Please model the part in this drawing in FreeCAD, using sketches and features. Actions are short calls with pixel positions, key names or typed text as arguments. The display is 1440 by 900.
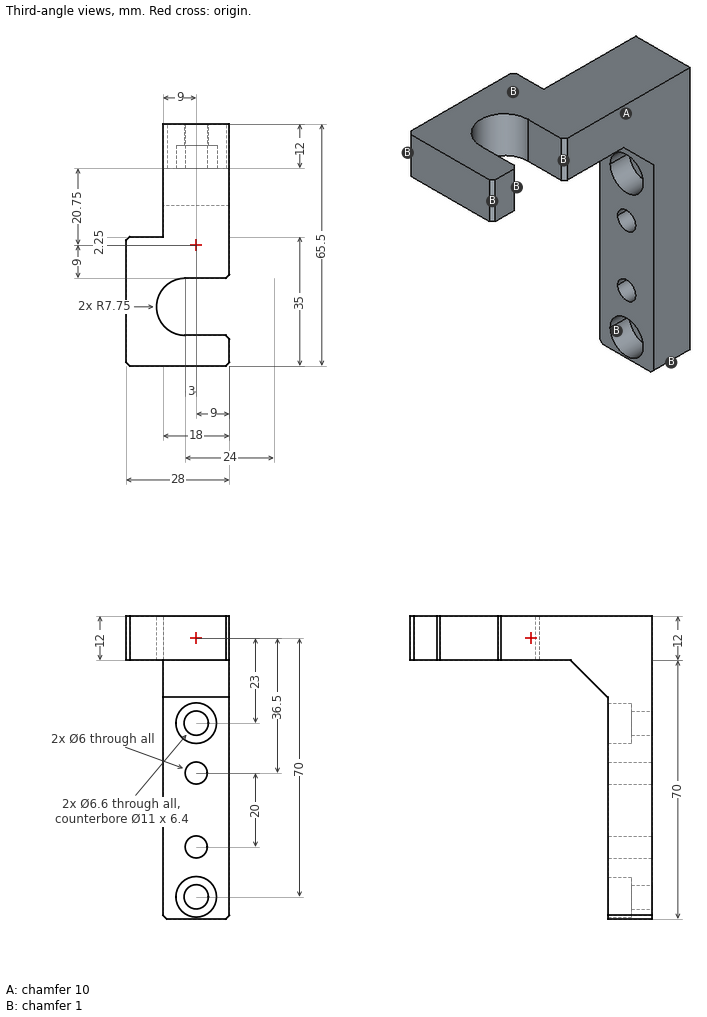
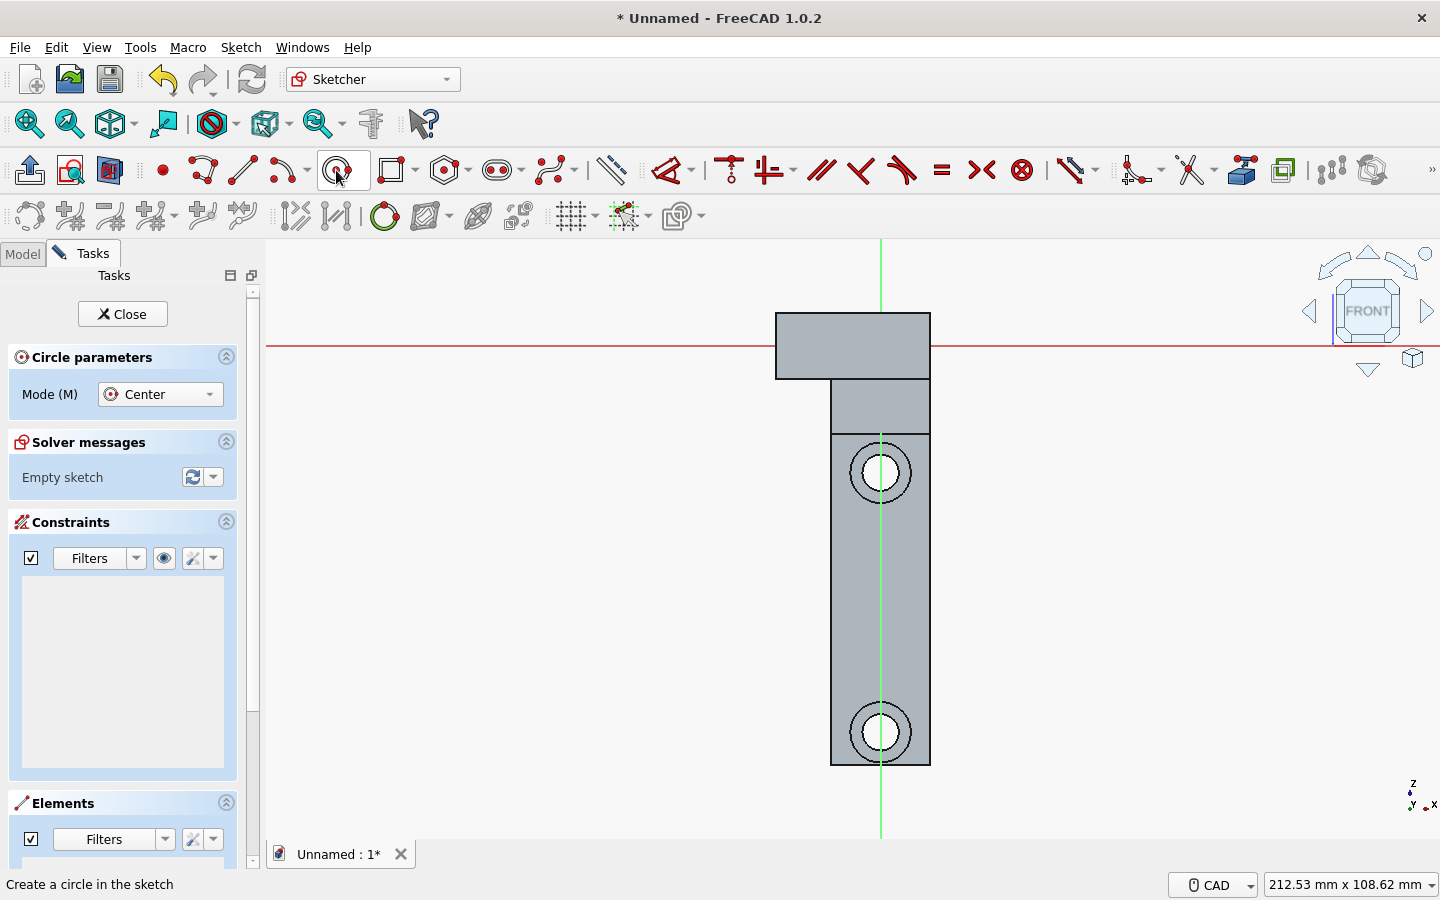
scroll(881, 547, up, 2)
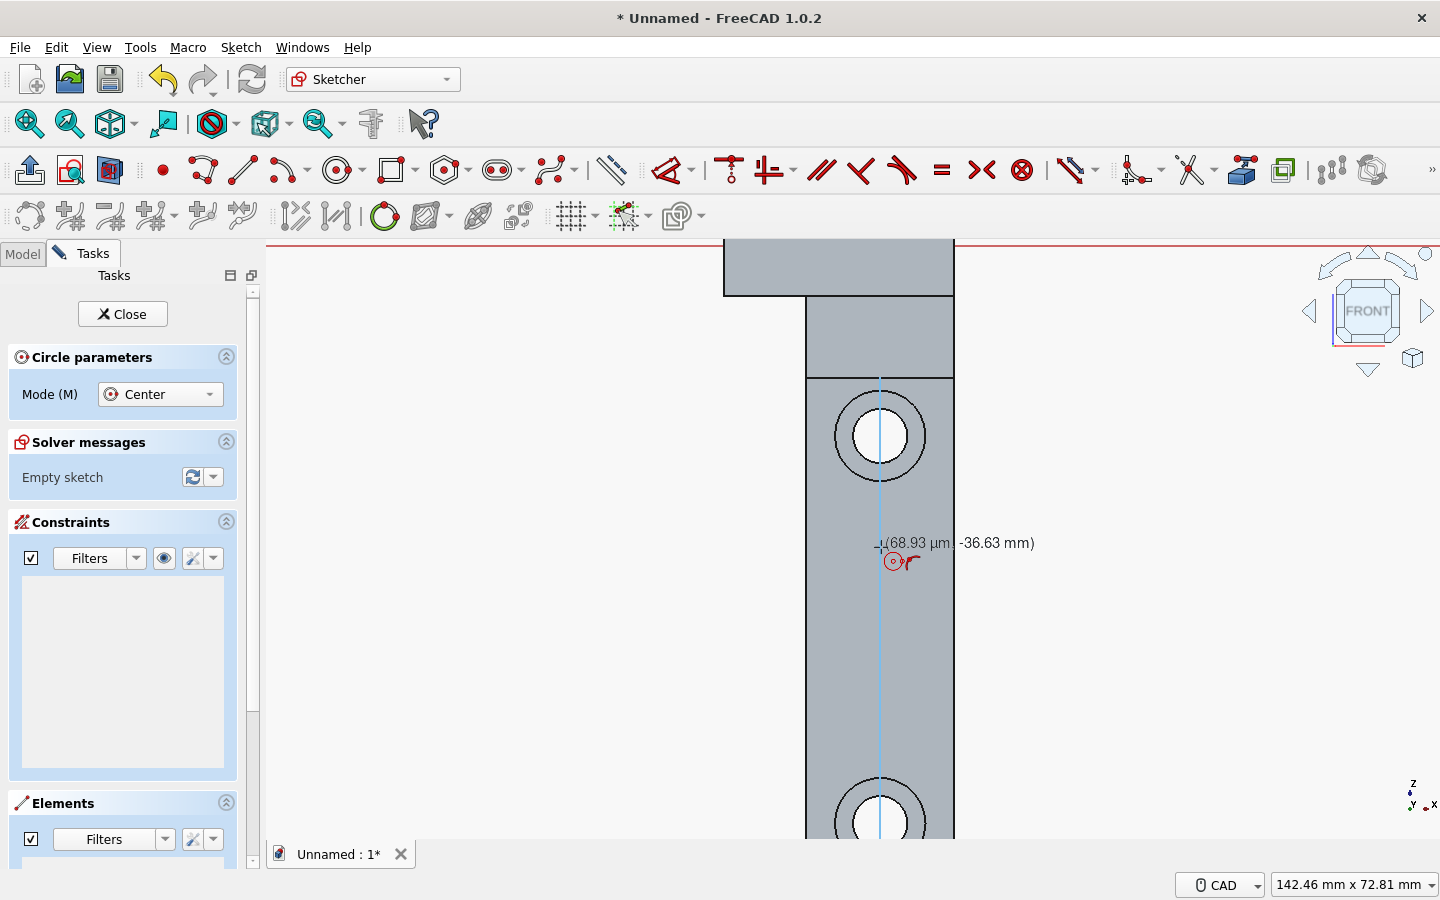
click(880, 547)
move(898, 530)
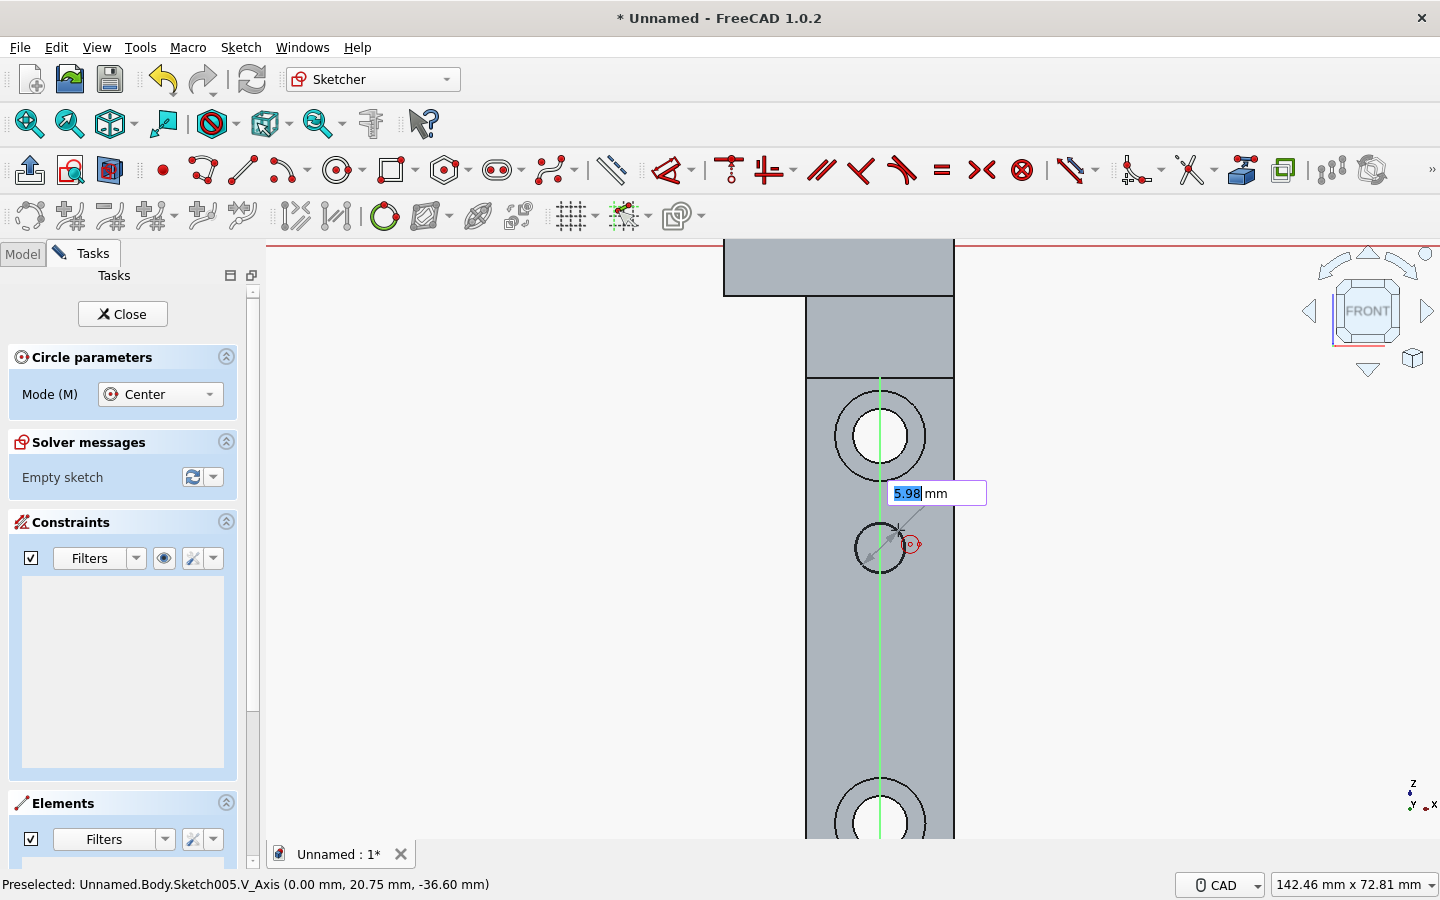
text(6)
key(Return)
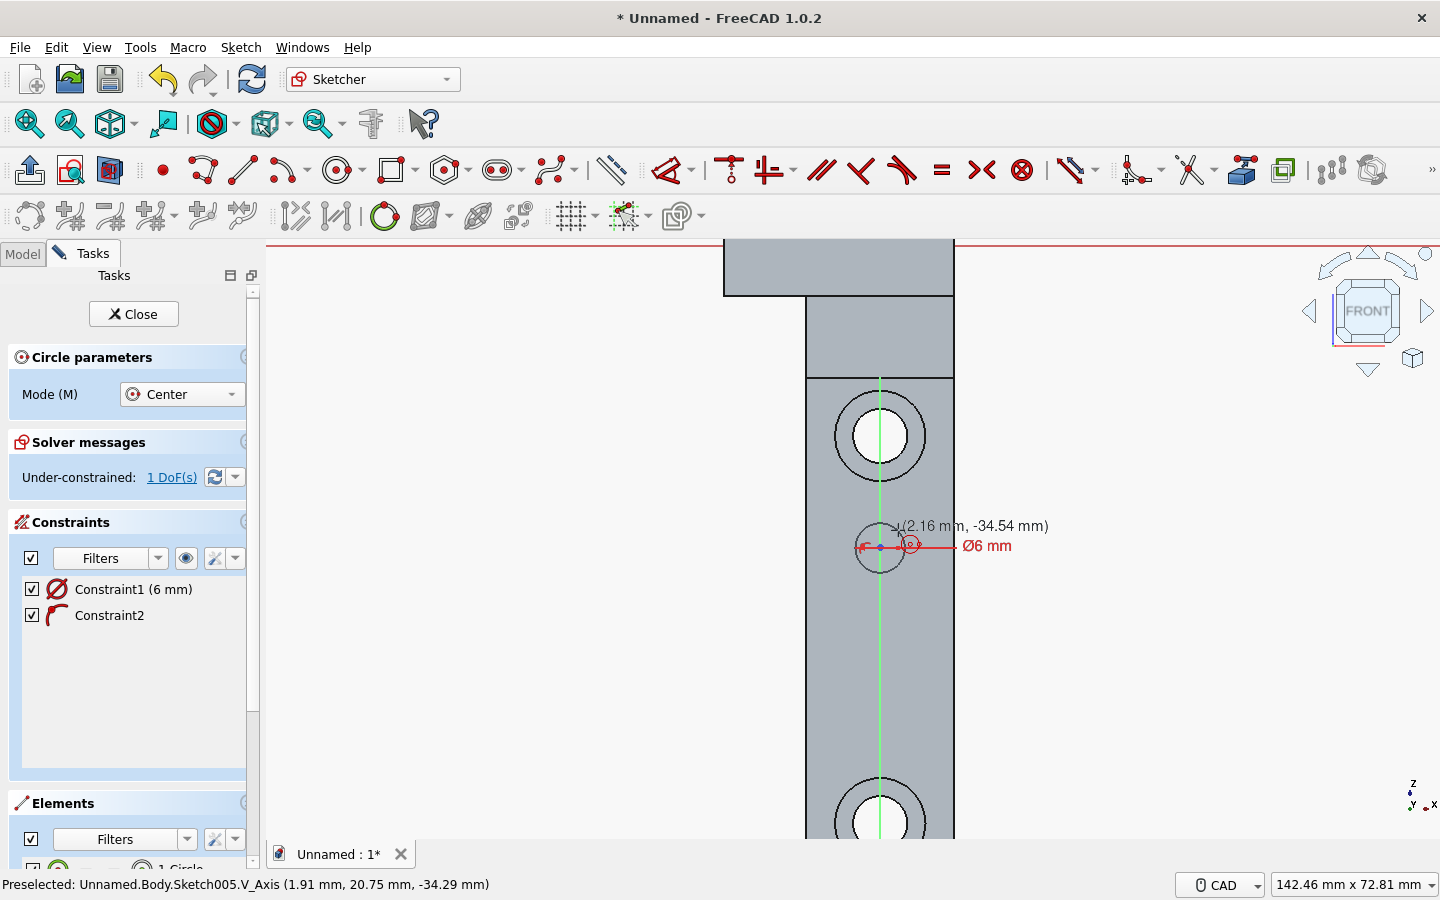
click(880, 712)
move(898, 695)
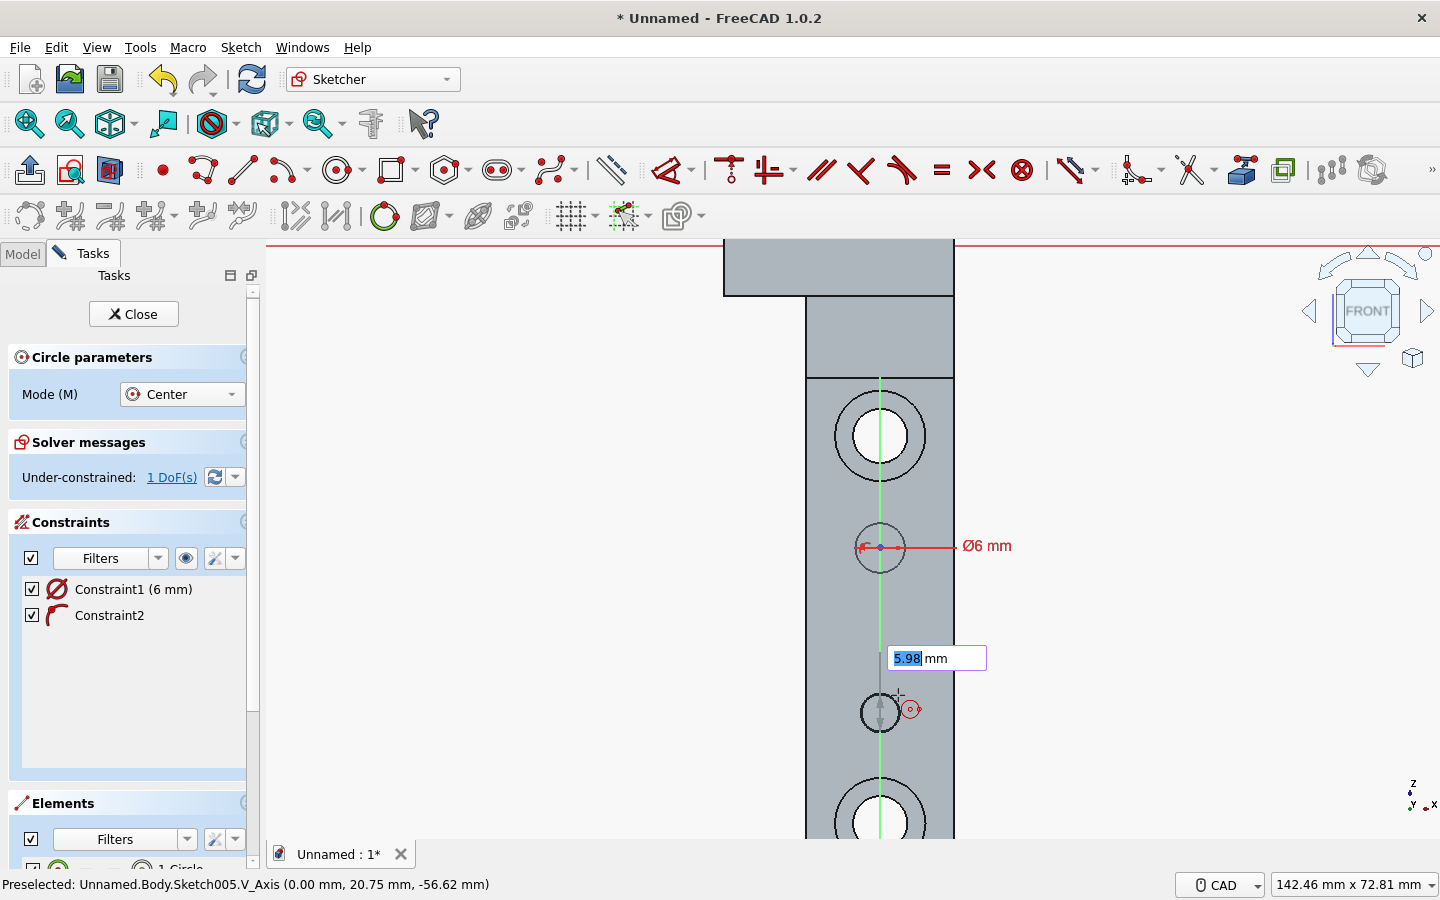
text(6)
key(Return)
key(Escape)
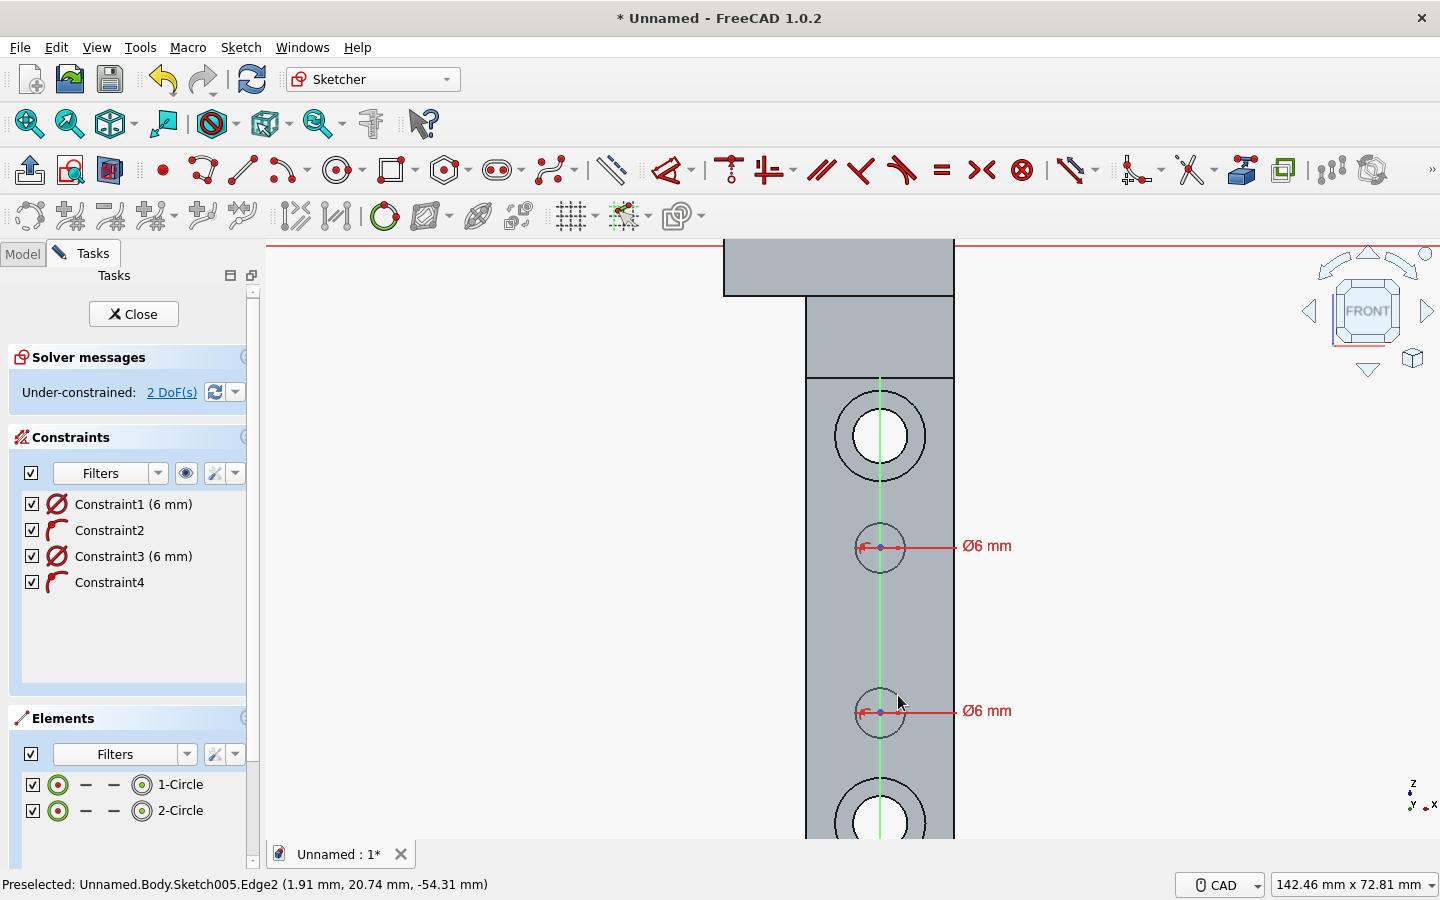
click(666, 170)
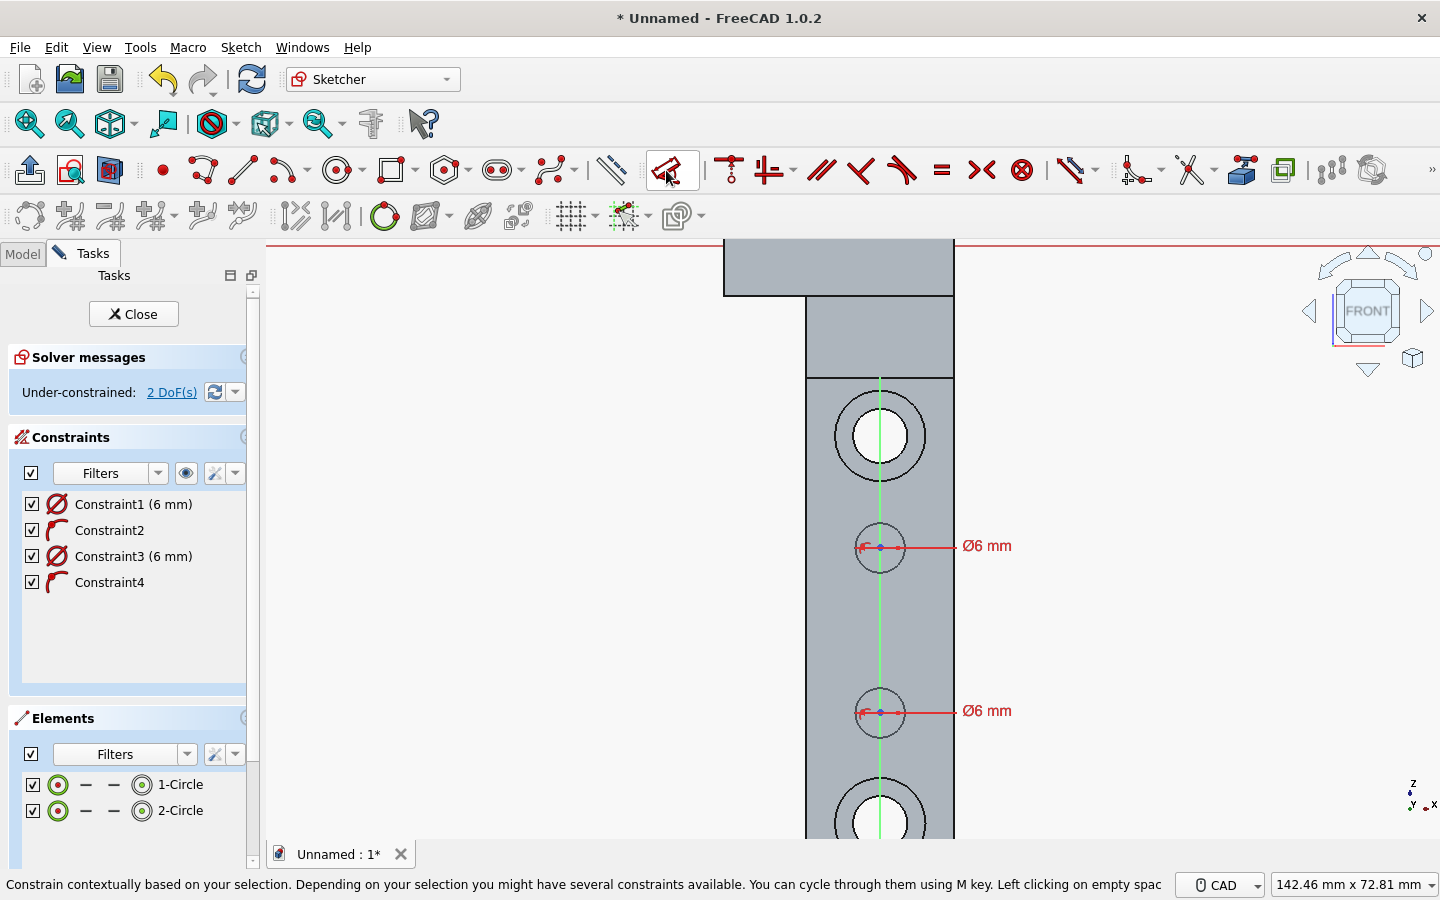
click(880, 548)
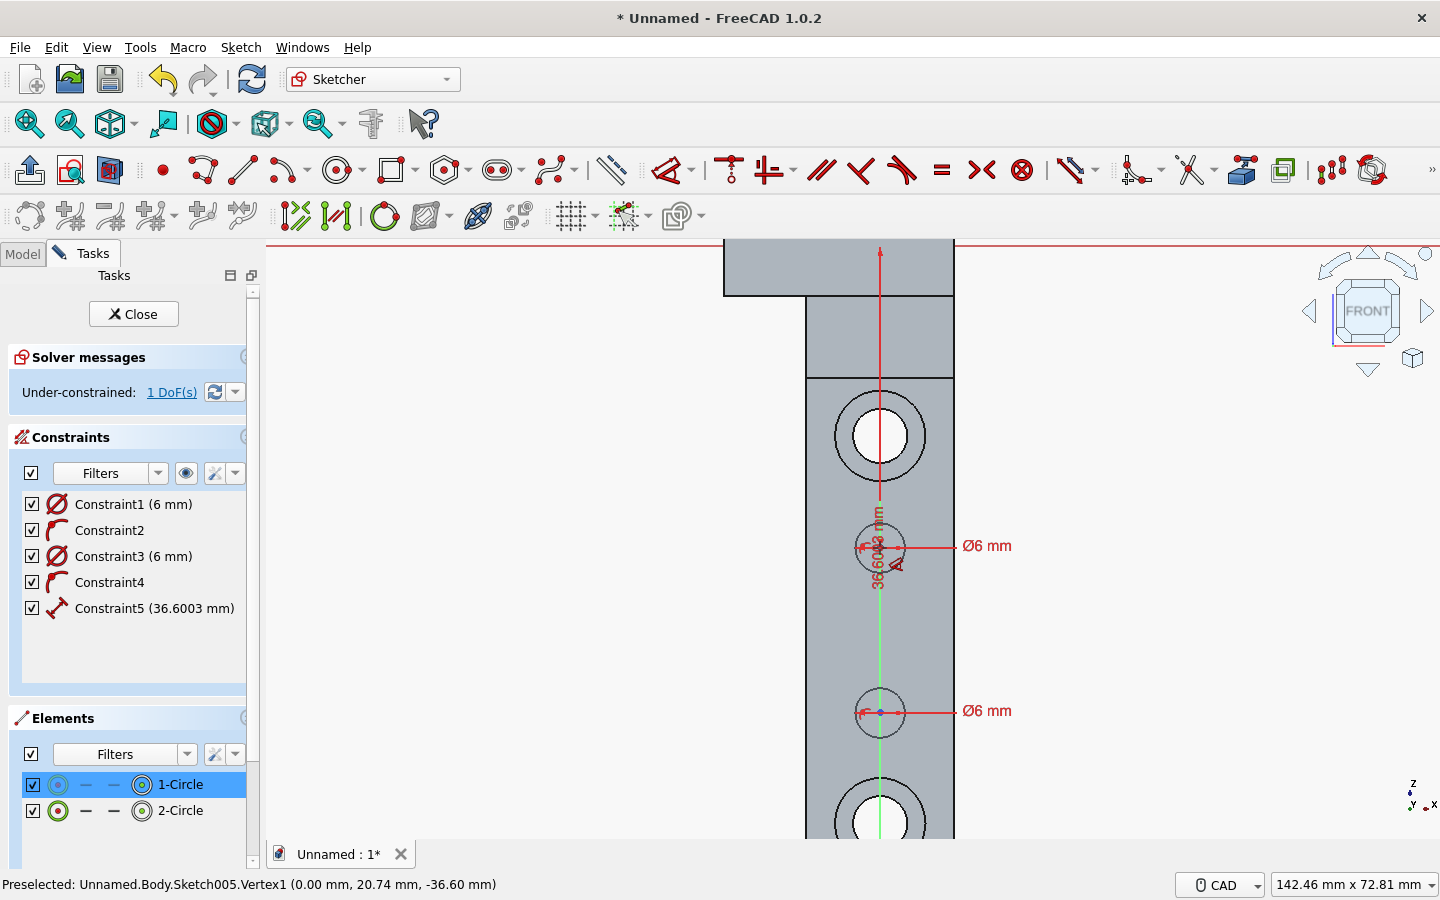
click(880, 713)
click(914, 630)